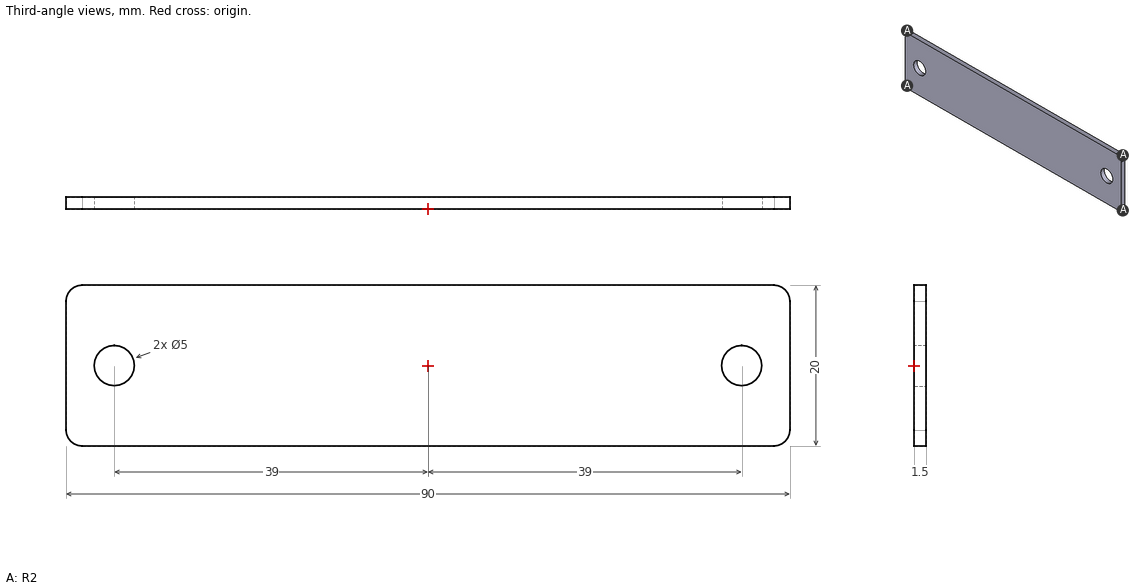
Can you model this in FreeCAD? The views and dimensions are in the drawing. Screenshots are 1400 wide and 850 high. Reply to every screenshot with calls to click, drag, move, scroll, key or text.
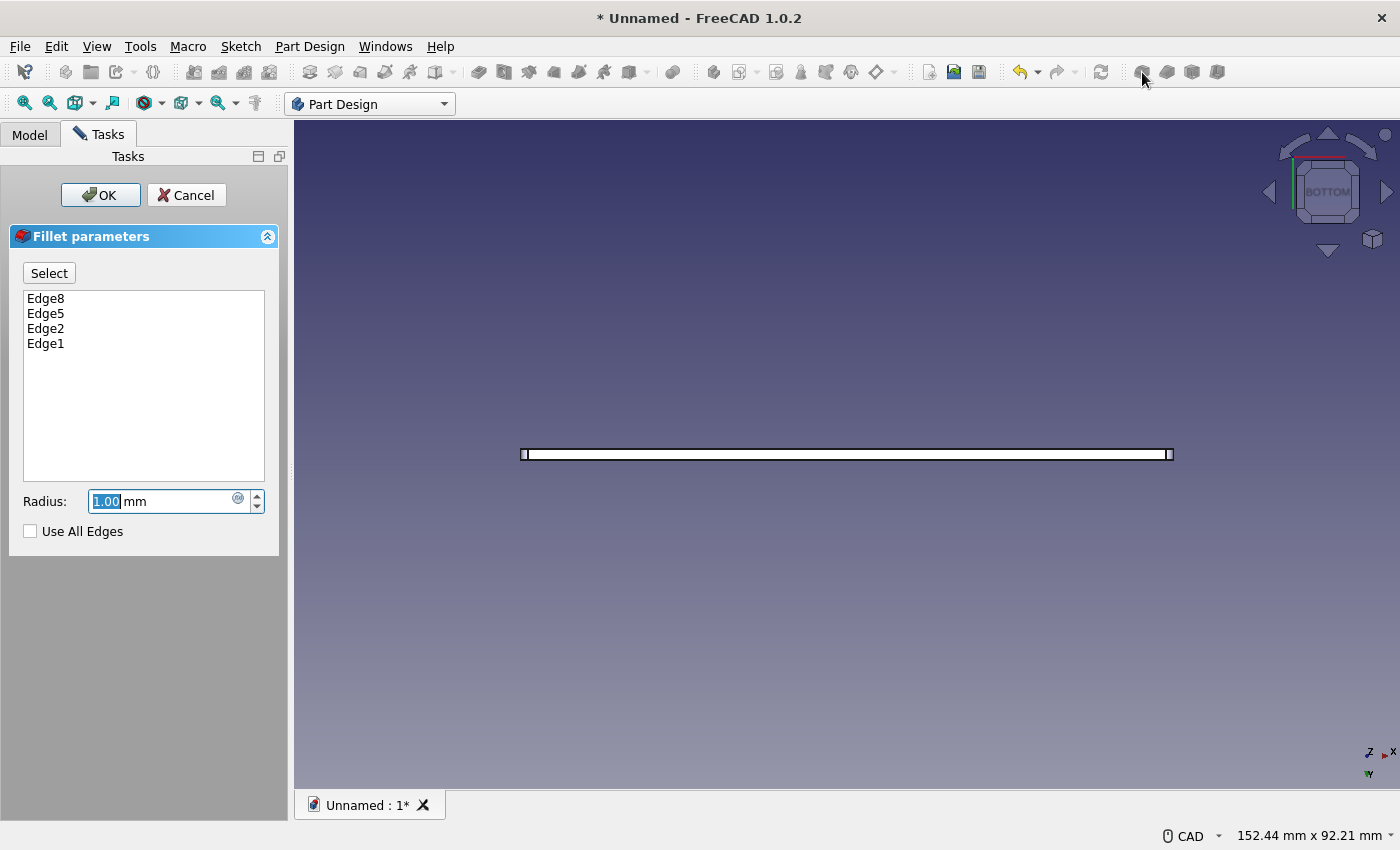
text(2)
key(Tab)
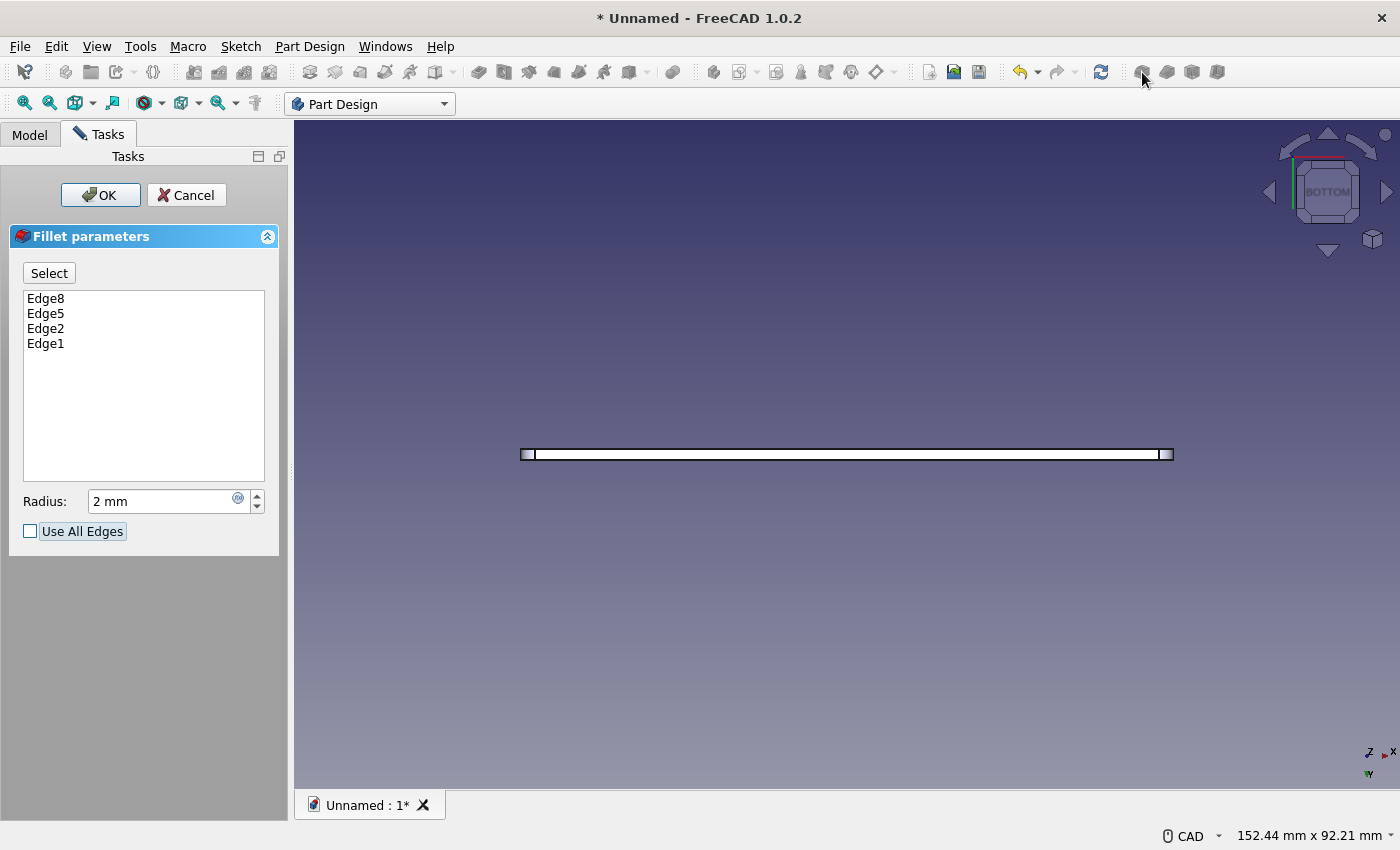
click(101, 195)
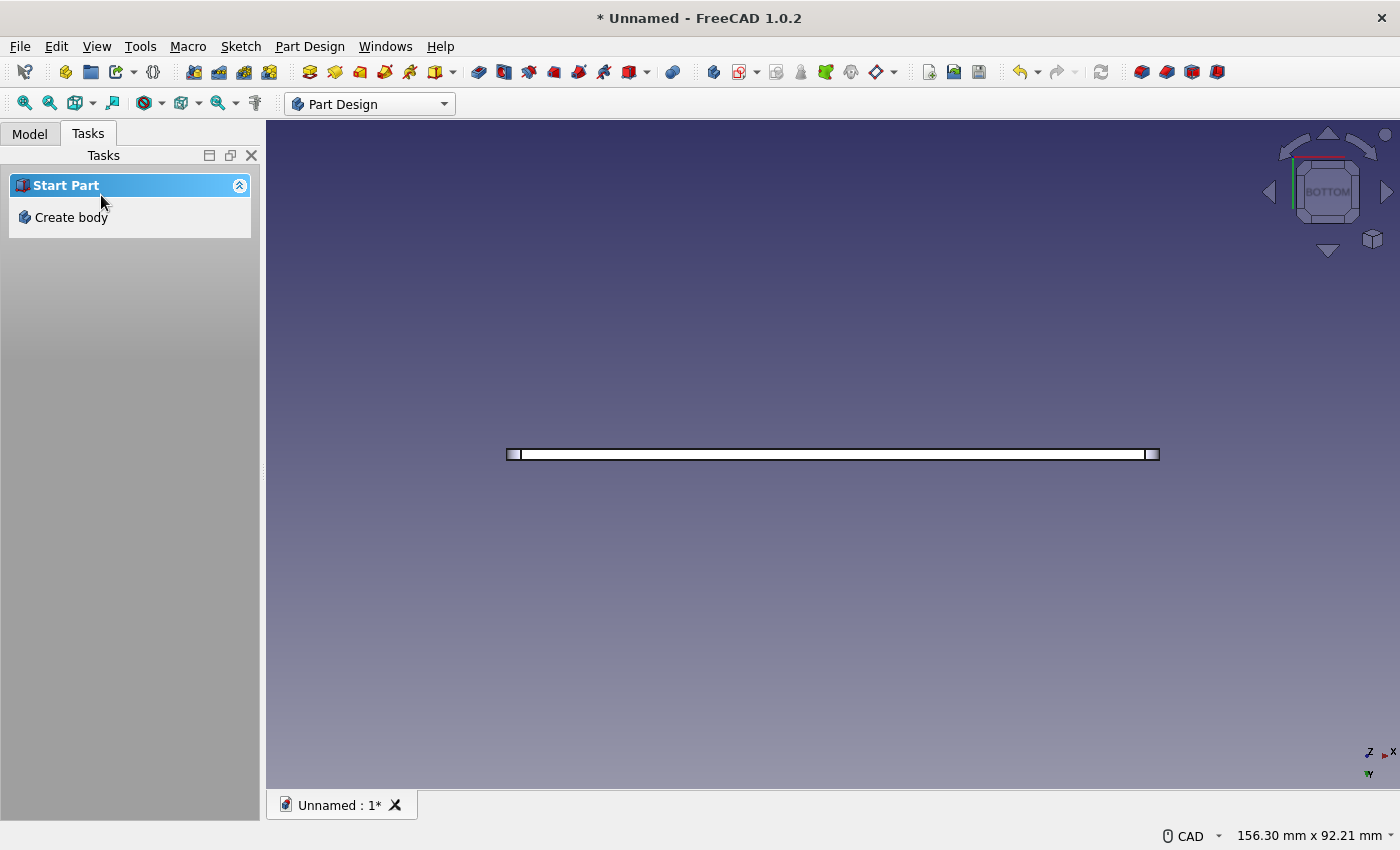
key(0)